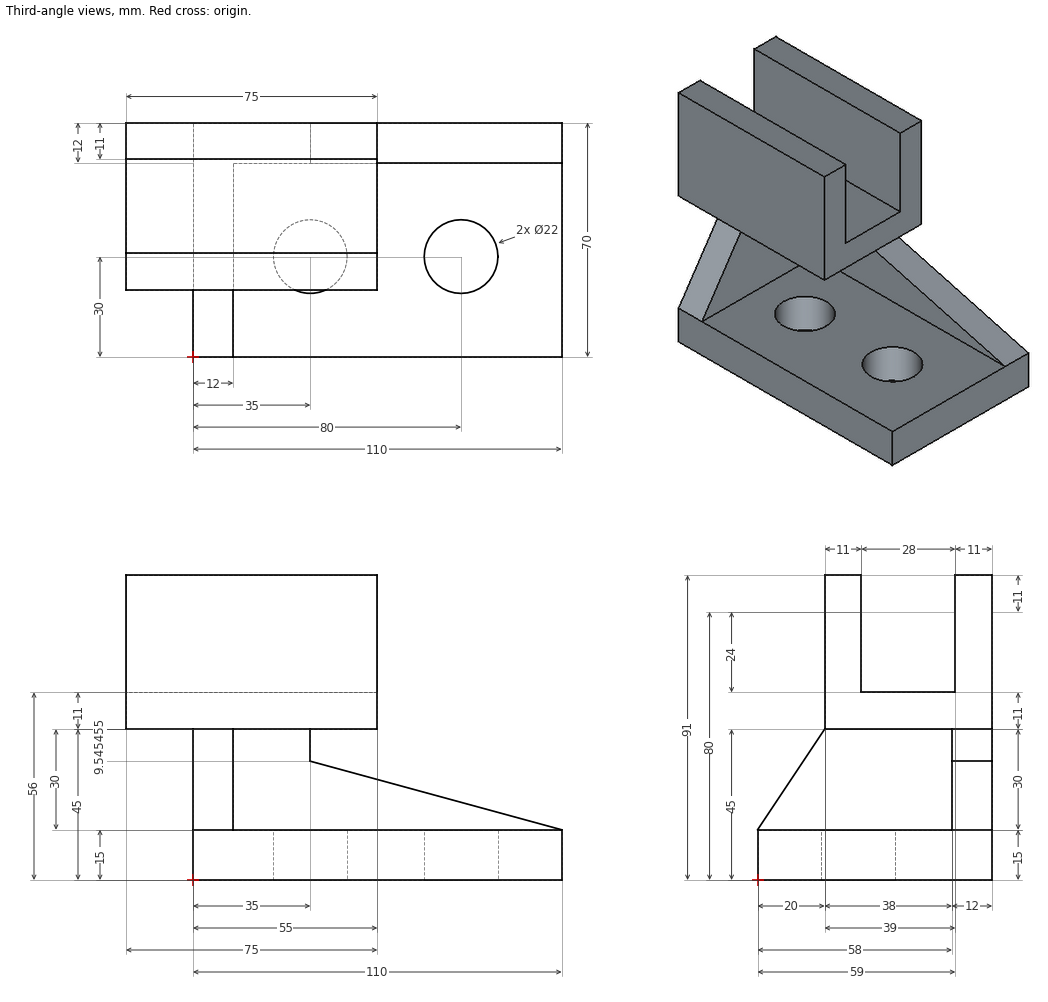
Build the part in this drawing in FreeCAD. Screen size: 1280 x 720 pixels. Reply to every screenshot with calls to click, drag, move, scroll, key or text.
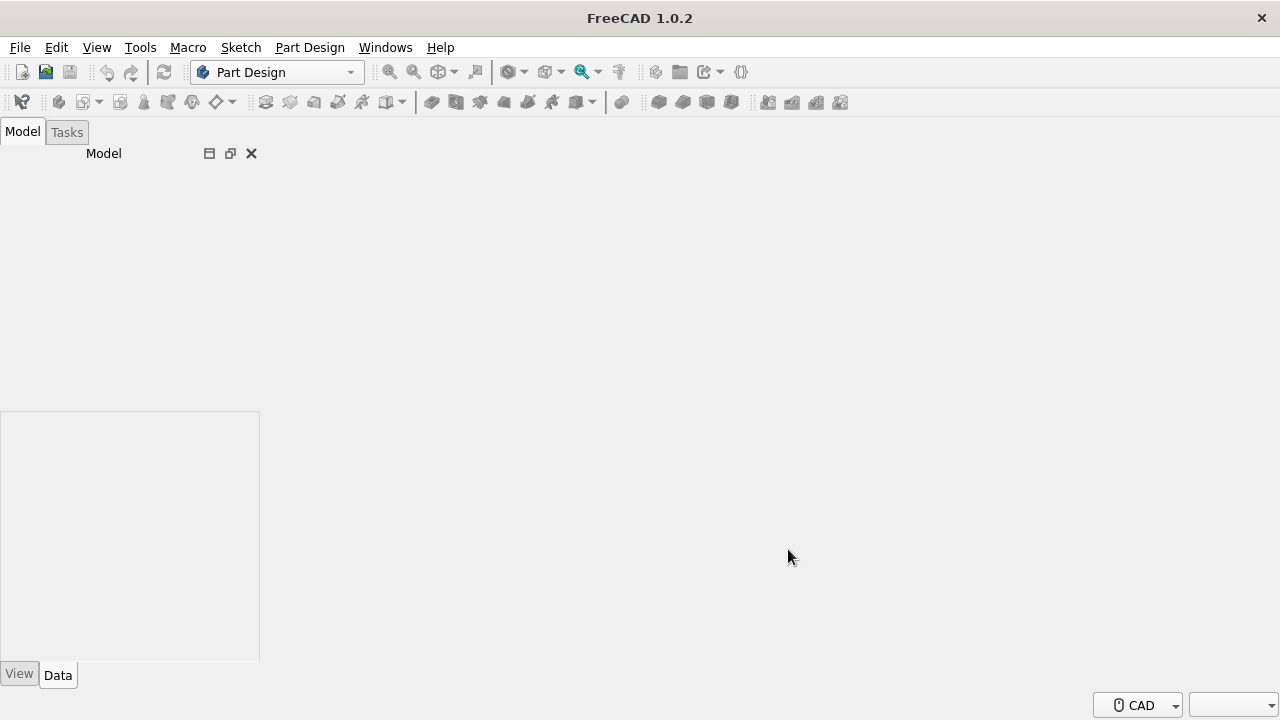
click(22, 72)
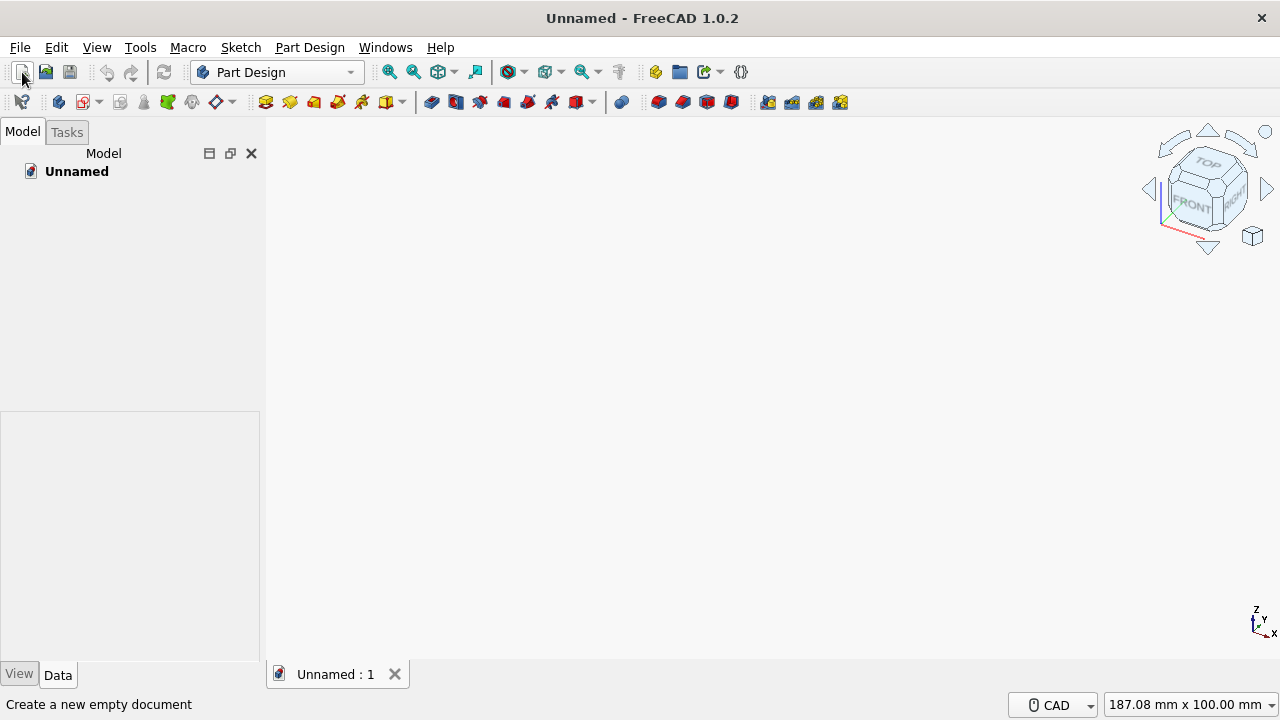
click(84, 102)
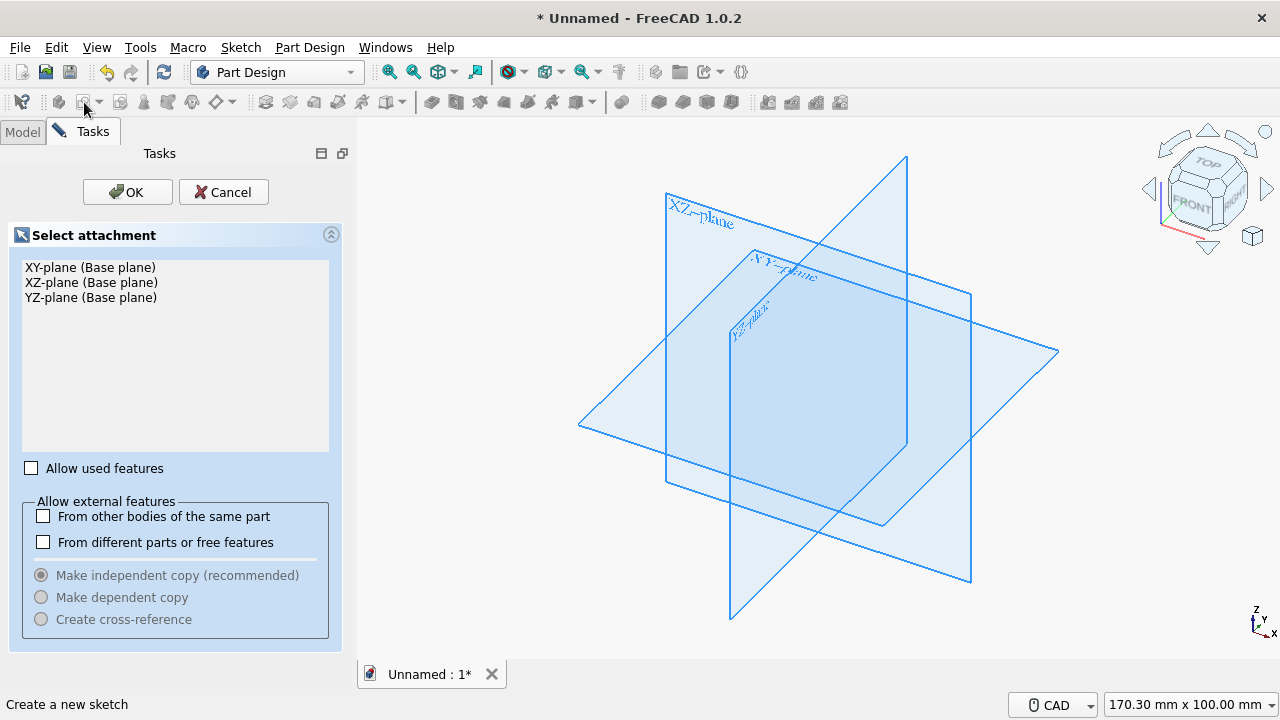
click(82, 268)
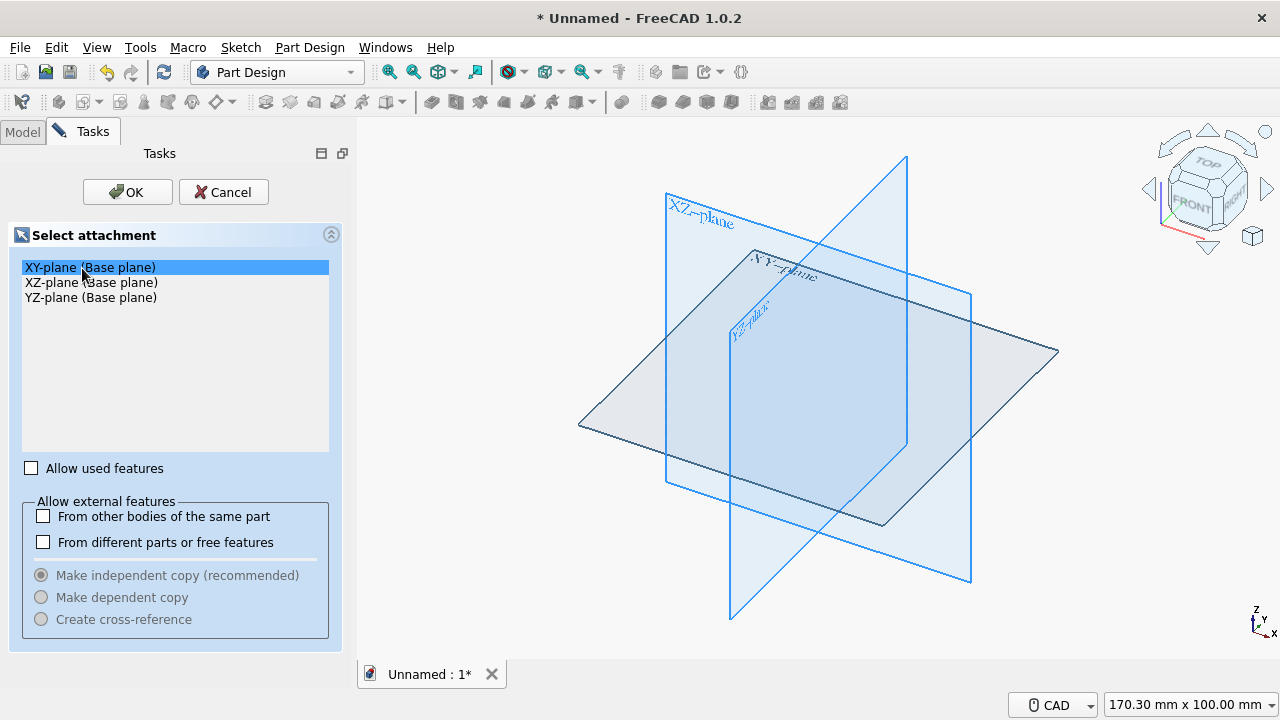
click(128, 192)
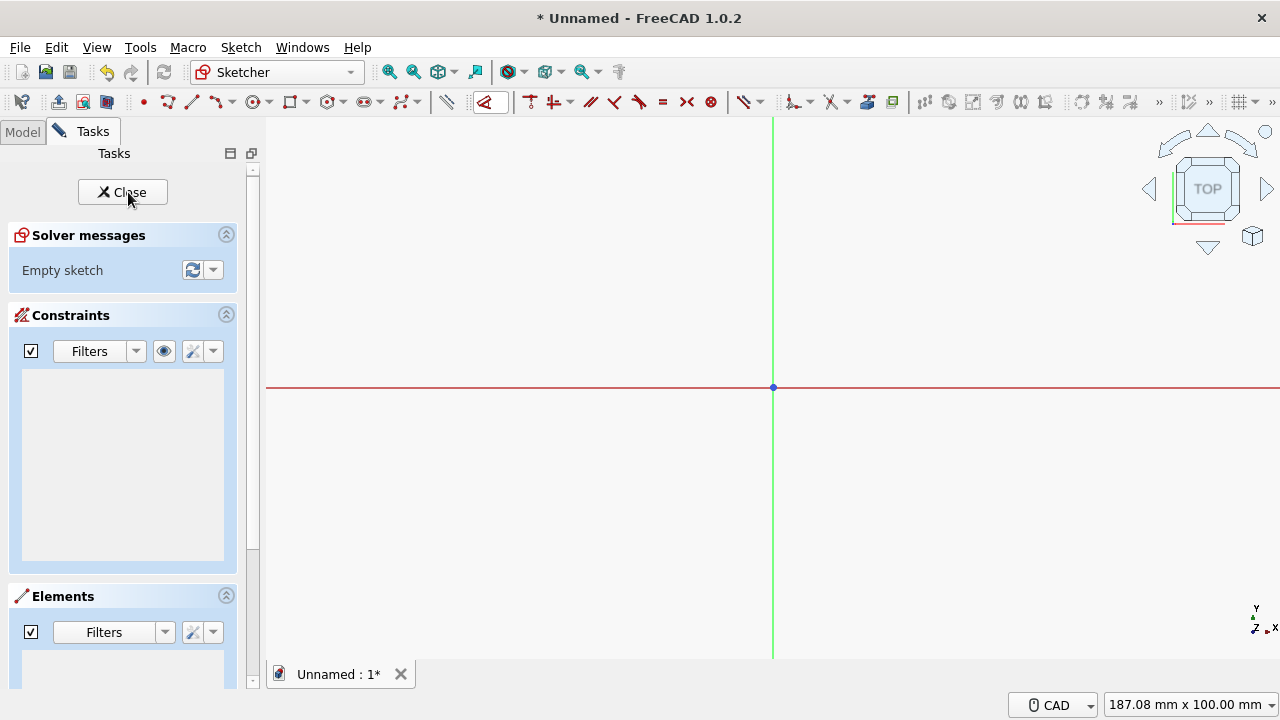
scroll(294, 631, down, 2)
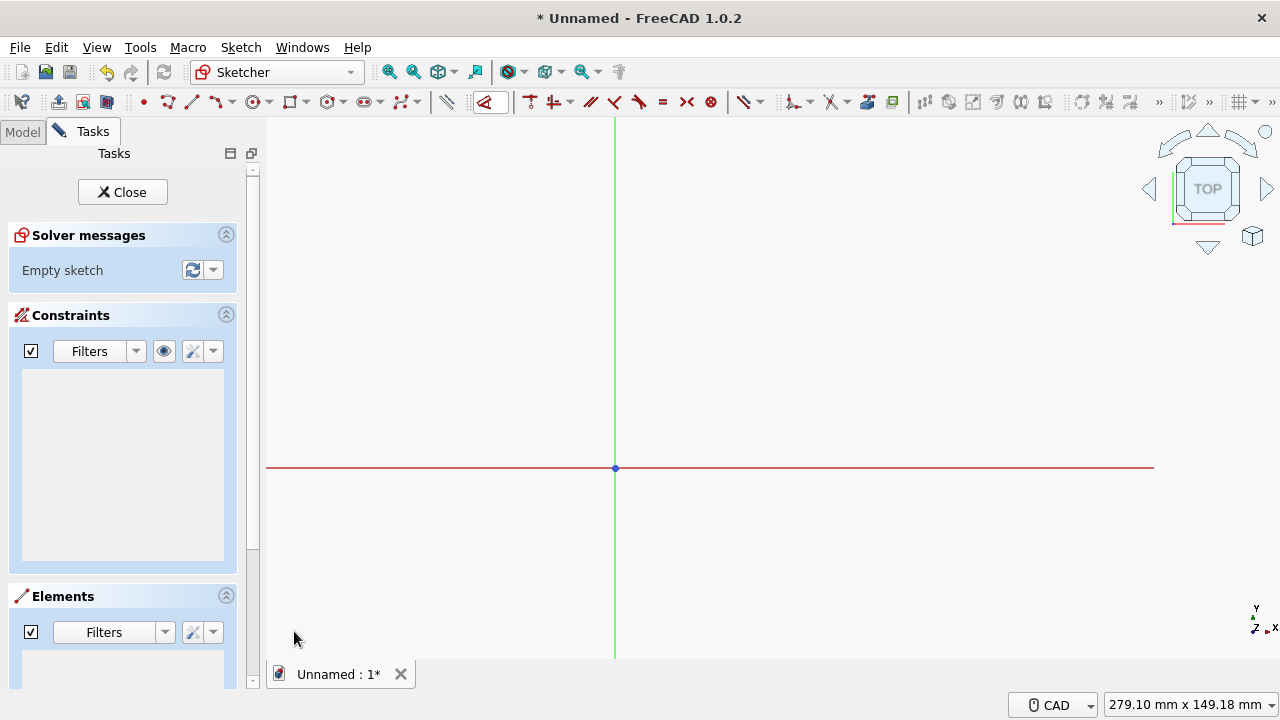
click(290, 102)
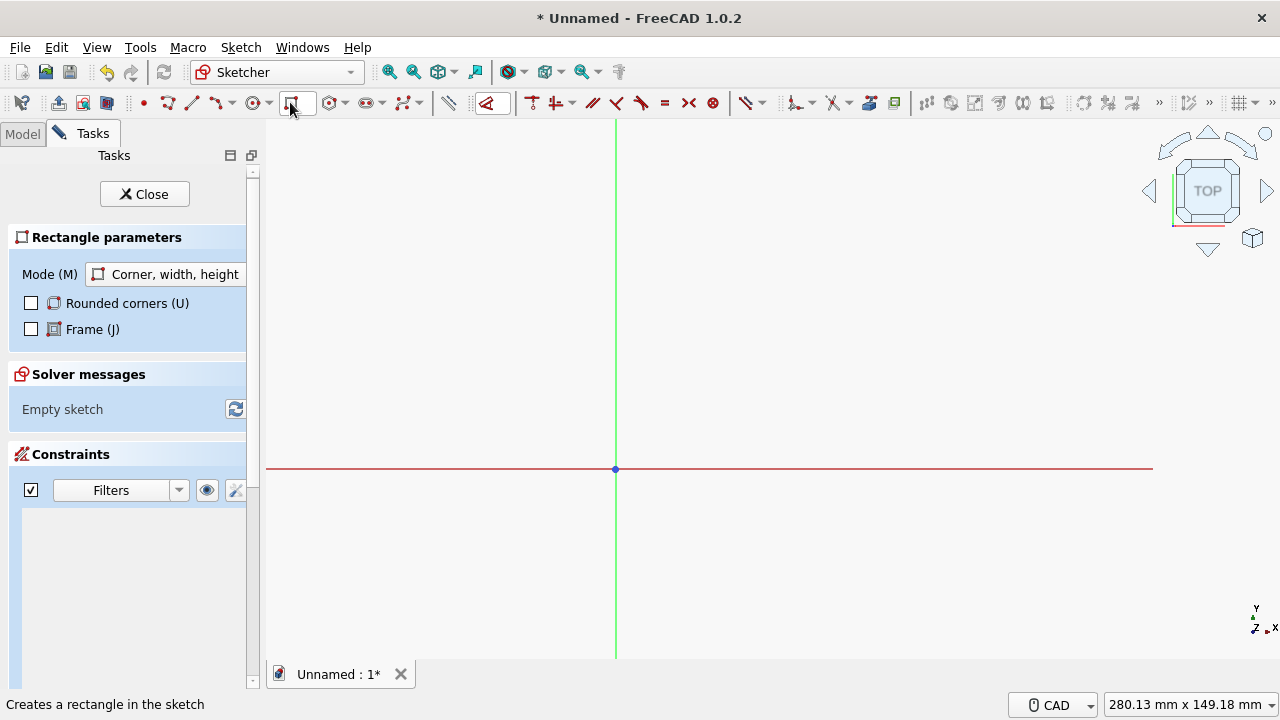
click(616, 469)
move(1014, 216)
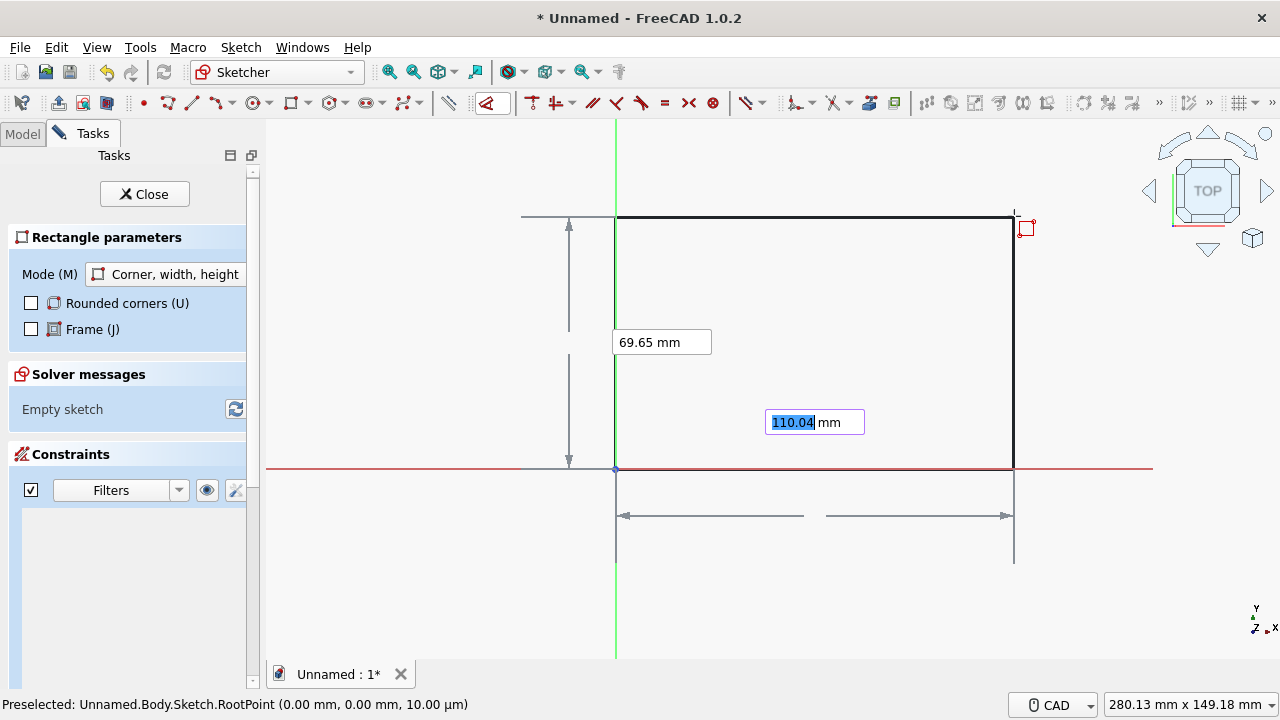
text(110)
key(Tab)
text(70)
key(Return)
key(Escape)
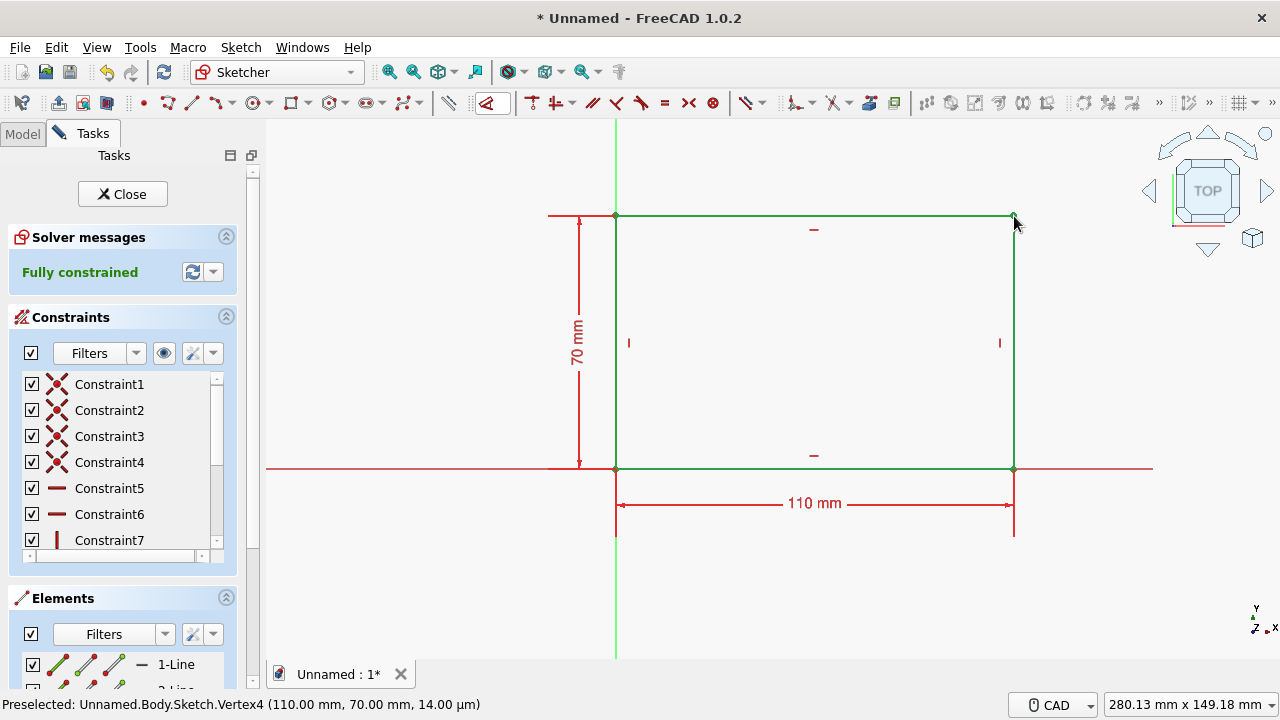
click(123, 194)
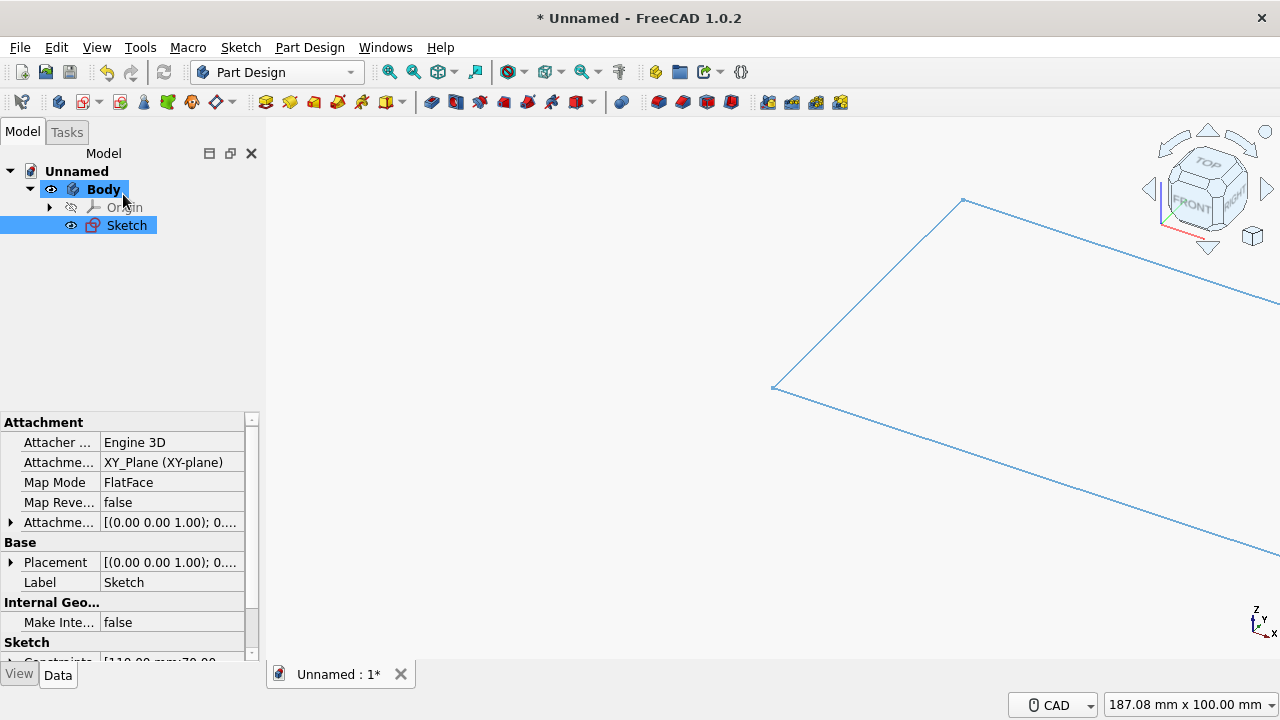
click(266, 102)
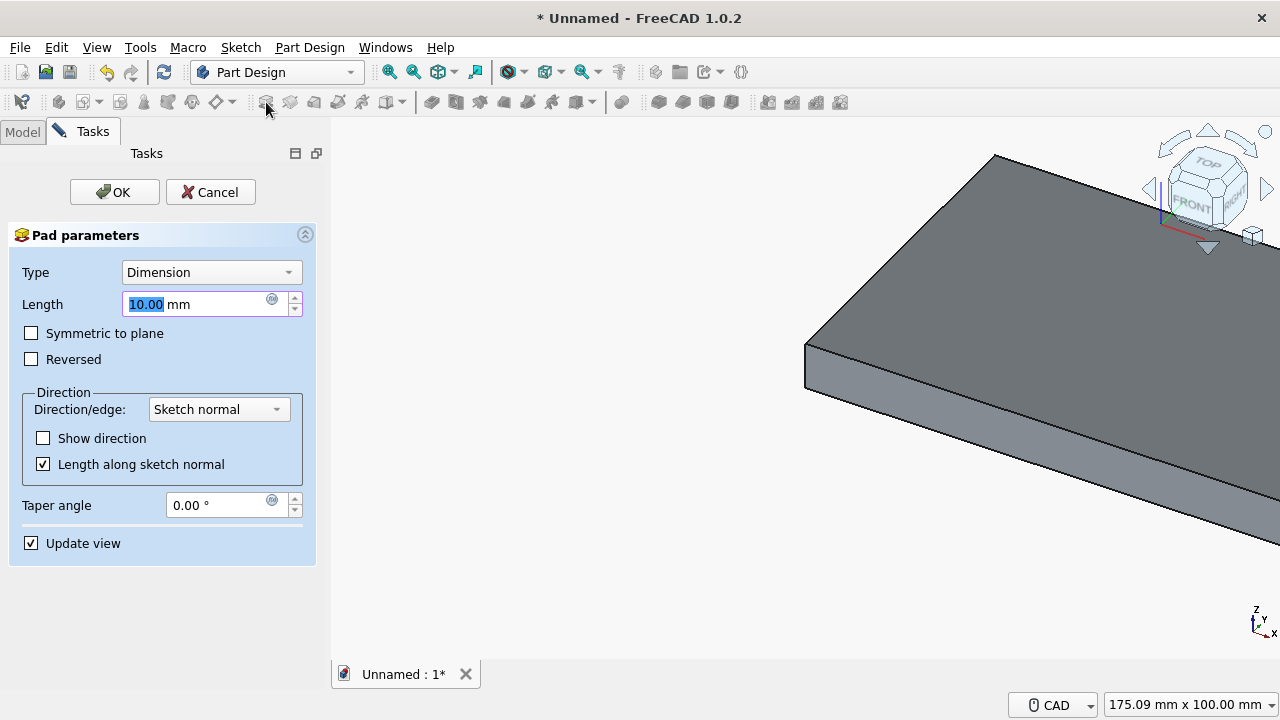
text(15)
key(Tab)